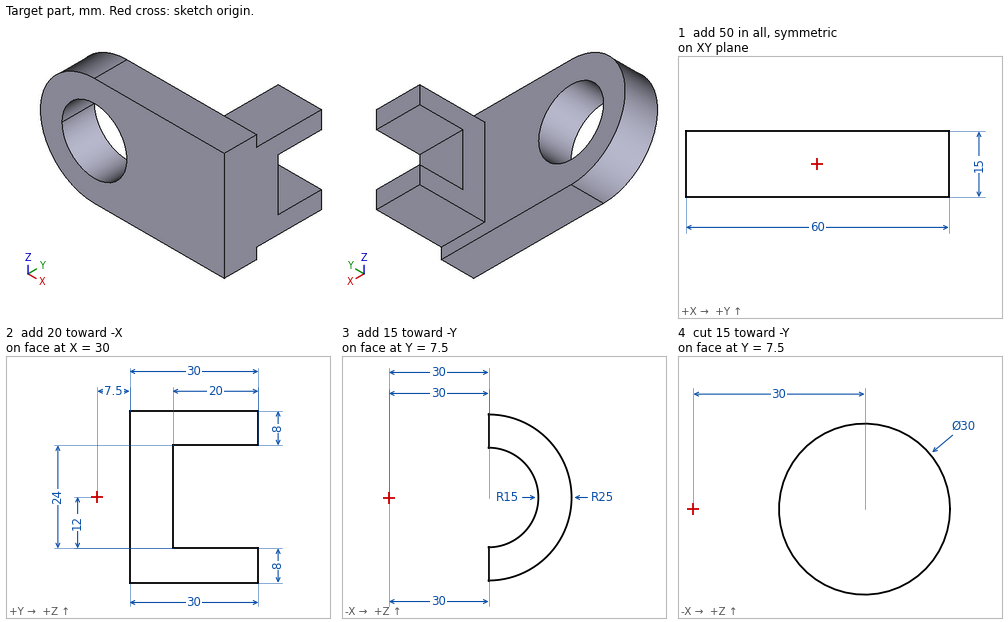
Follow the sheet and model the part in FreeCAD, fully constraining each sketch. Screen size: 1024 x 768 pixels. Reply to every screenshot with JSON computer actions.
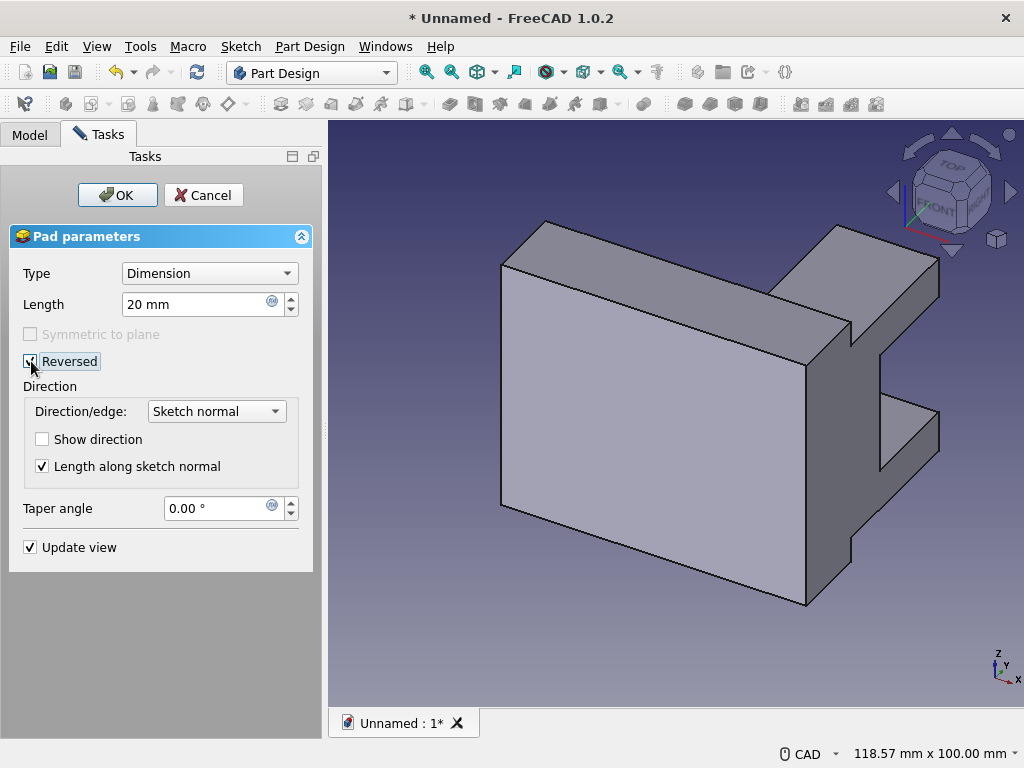
{"action": "left_click", "coordinate": [118, 195]}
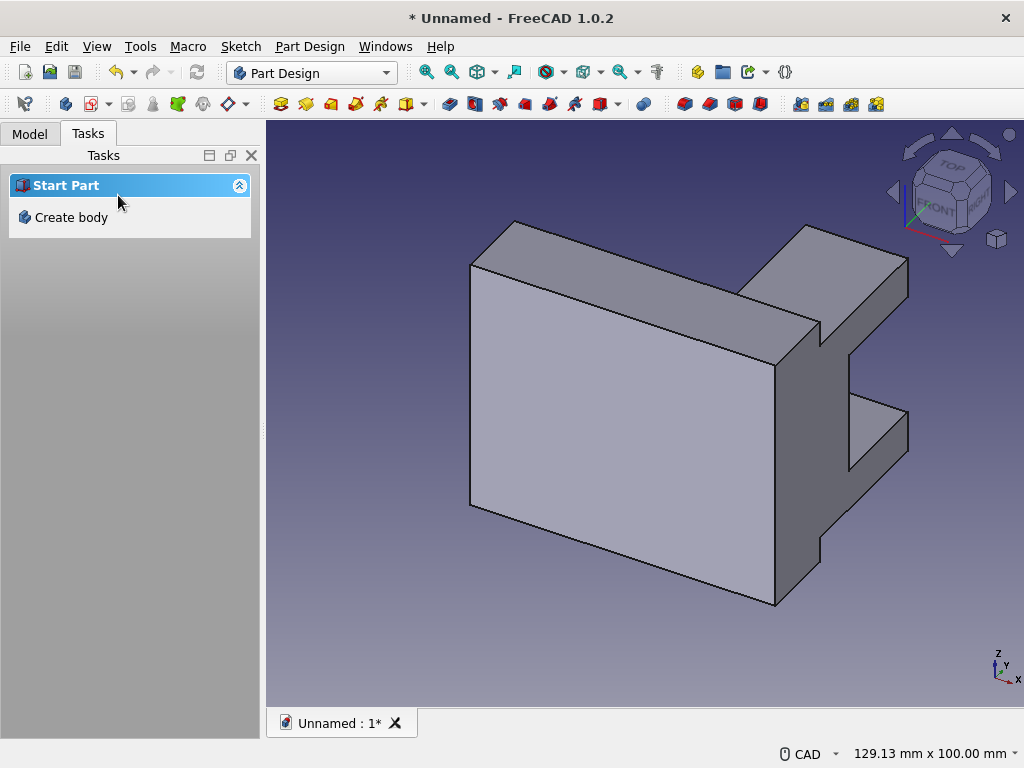
{"action": "key", "text": "4"}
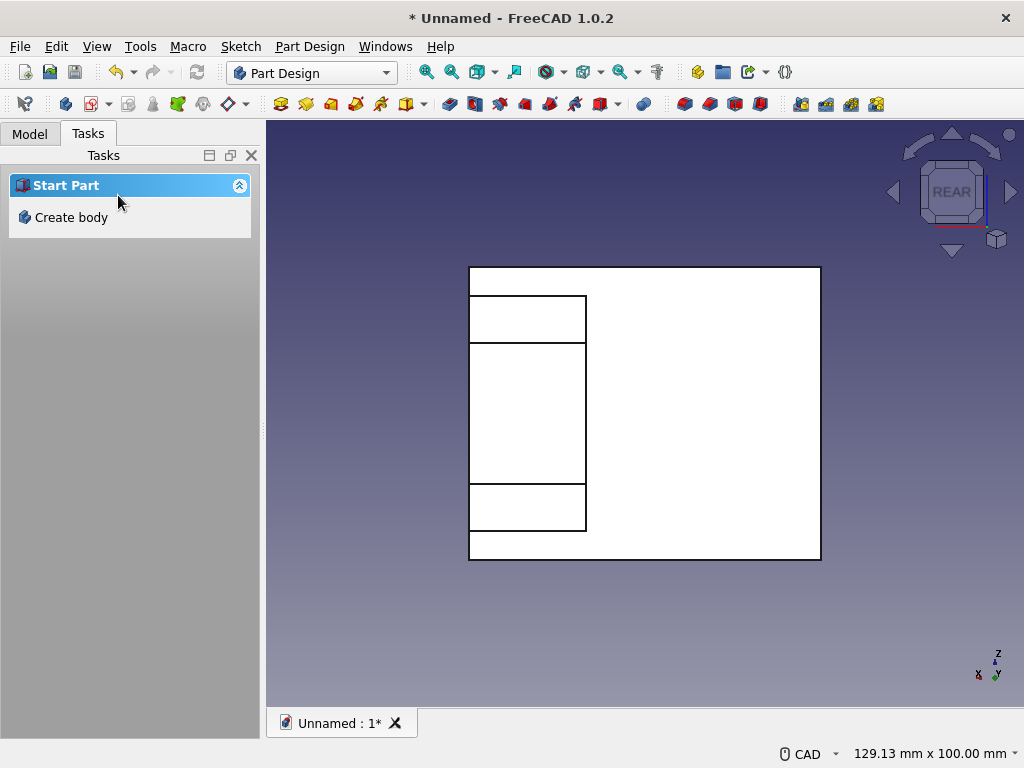
{"action": "left_click", "coordinate": [695, 412]}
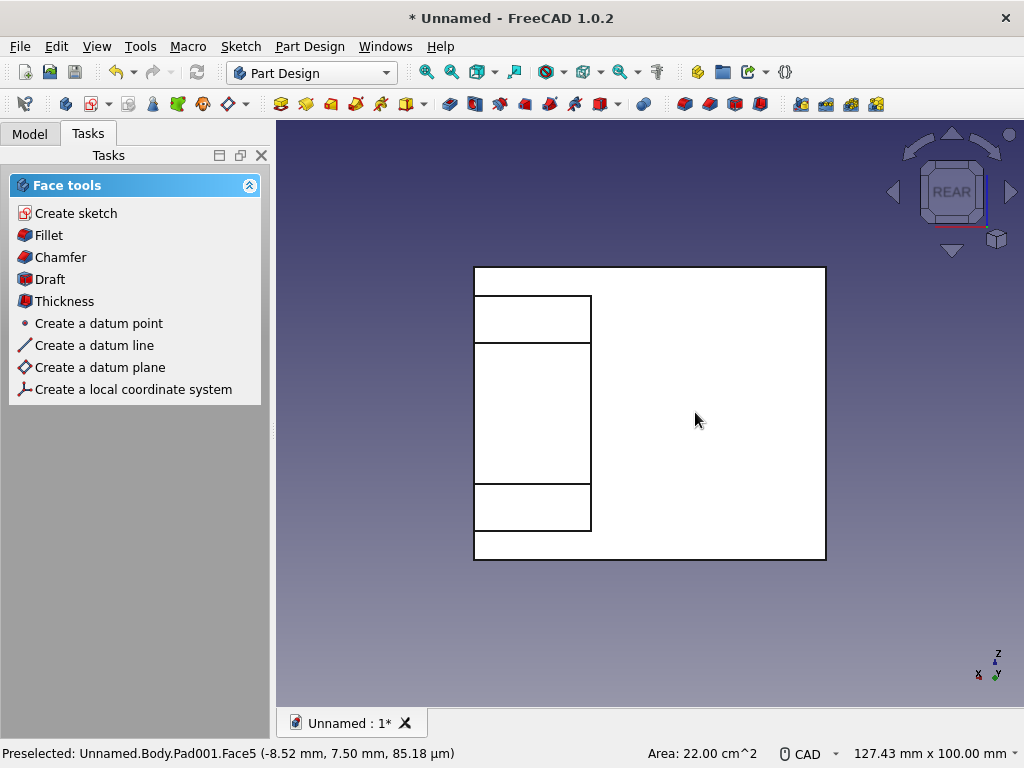
{"action": "left_click", "coordinate": [90, 104]}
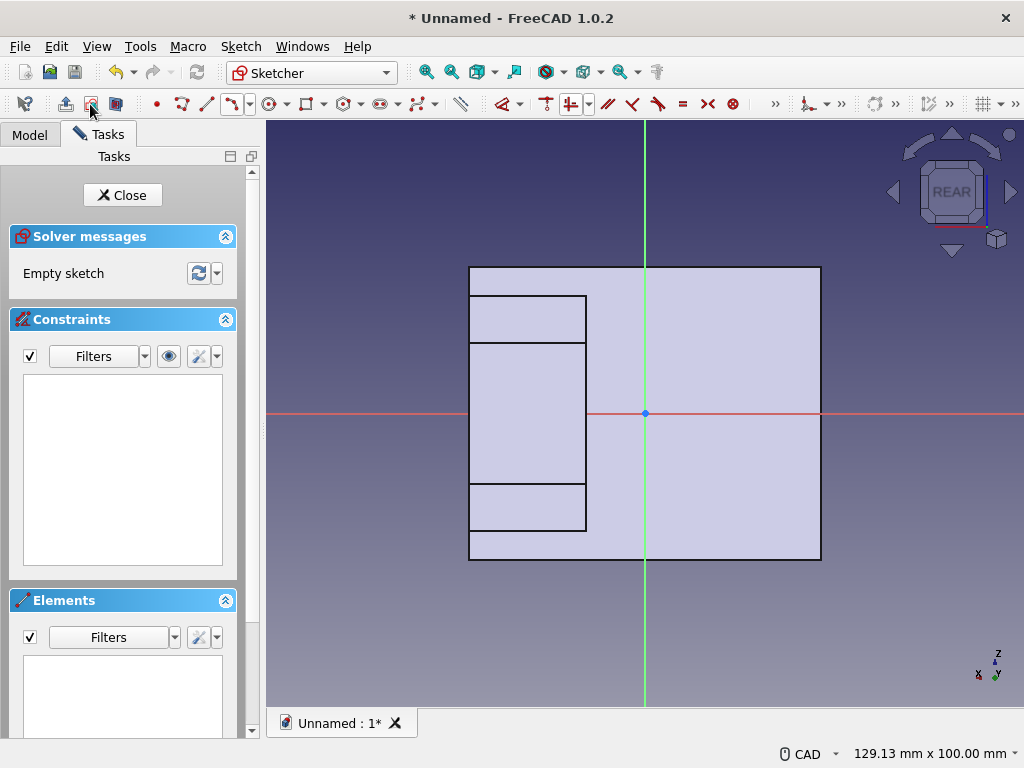
{"action": "scroll", "coordinate": [294, 414], "scroll_direction": "down", "scroll_amount": 2}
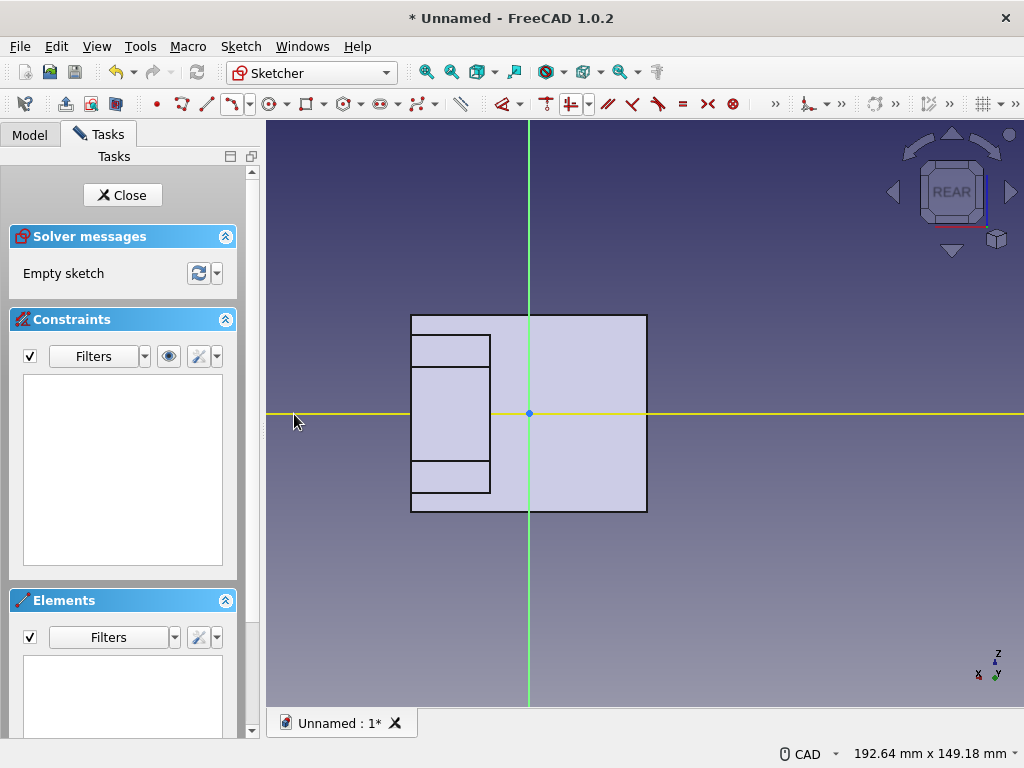
{"action": "scroll", "coordinate": [712, 414], "scroll_direction": "up", "scroll_amount": 3}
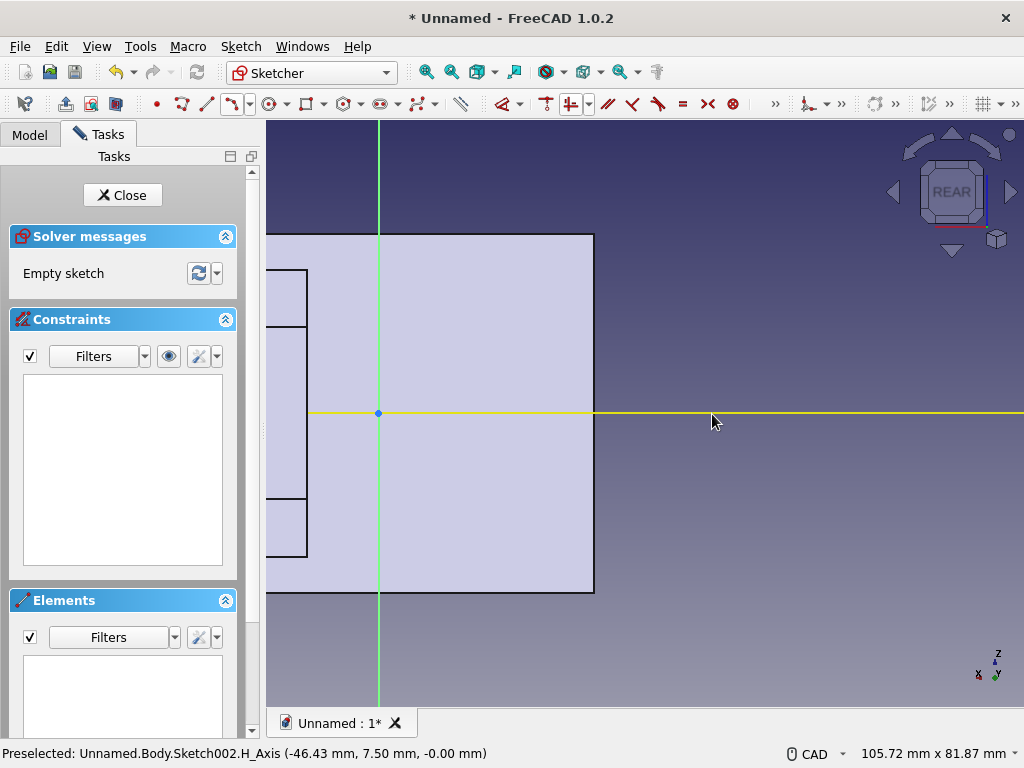
{"action": "key", "text": "g l"}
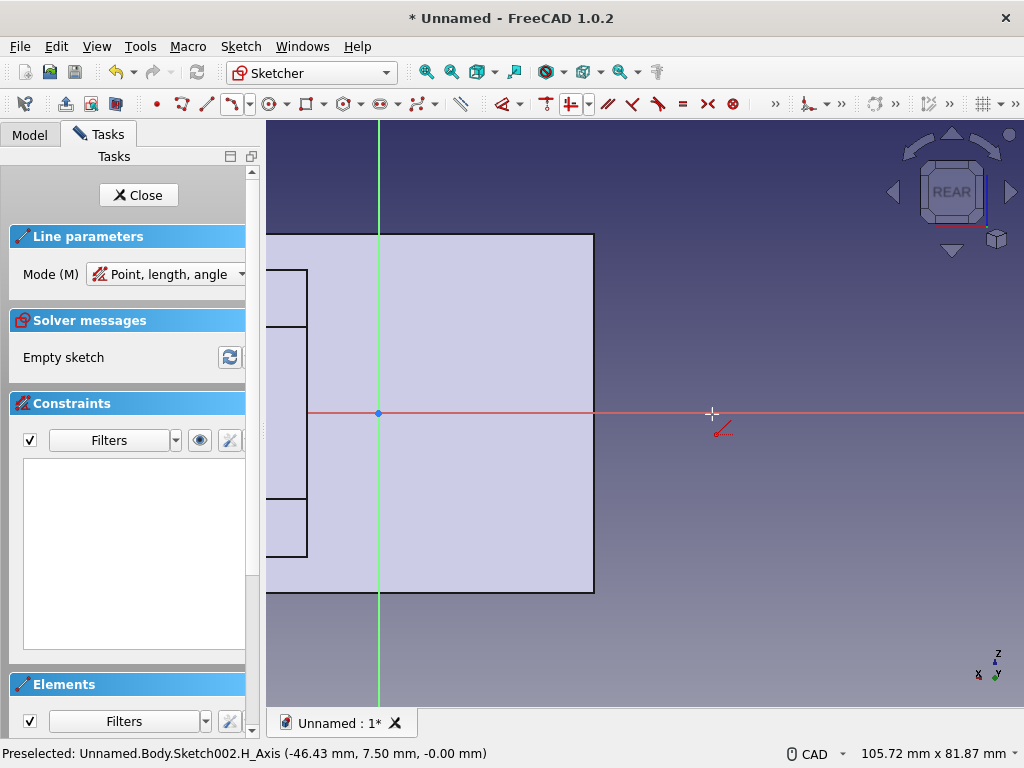
{"action": "left_click", "coordinate": [594, 521]}
{"action": "left_click", "coordinate": [594, 593]}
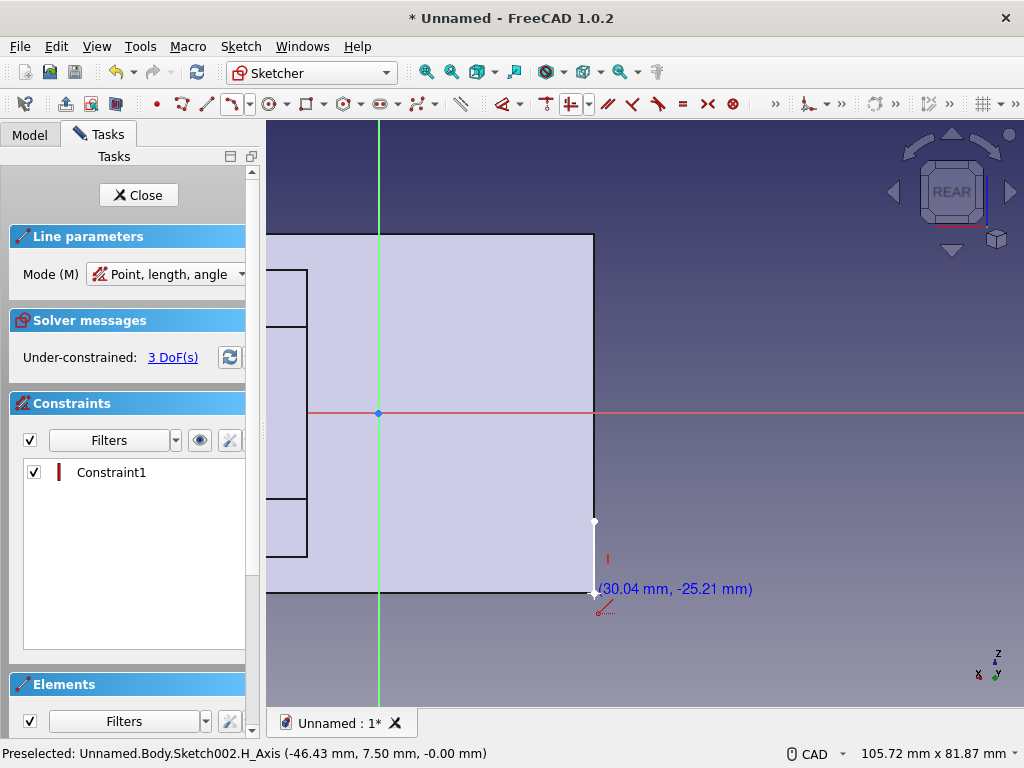
{"action": "left_click", "coordinate": [594, 234]}
{"action": "left_click", "coordinate": [594, 306]}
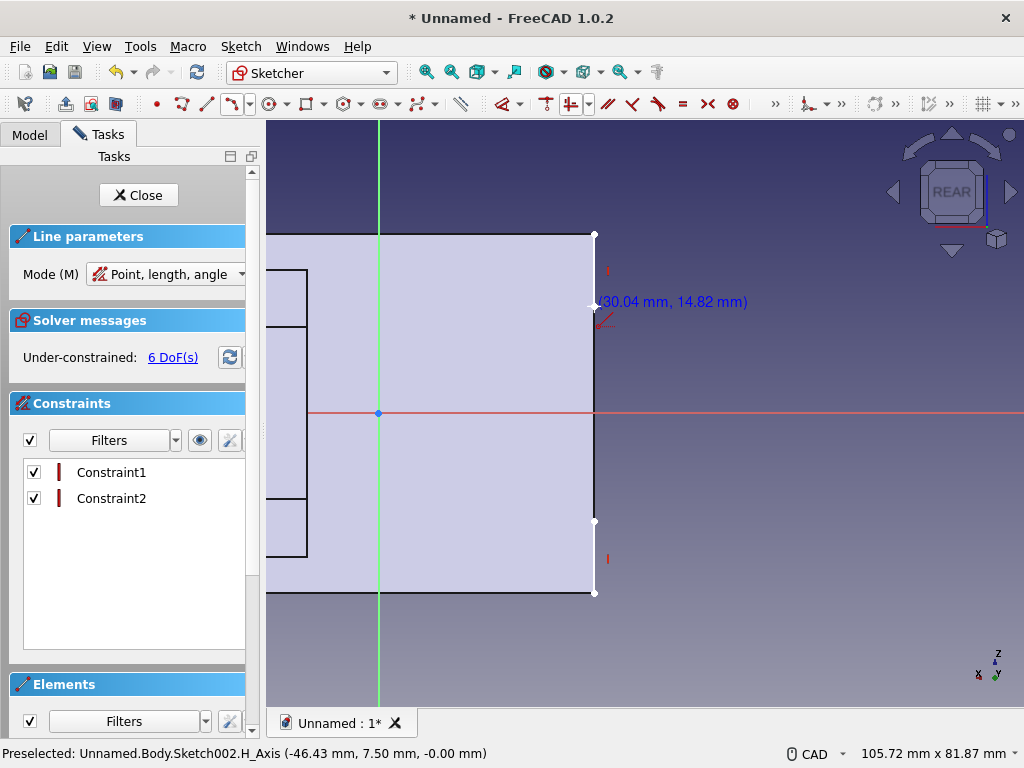
{"action": "left_click", "coordinate": [232, 104]}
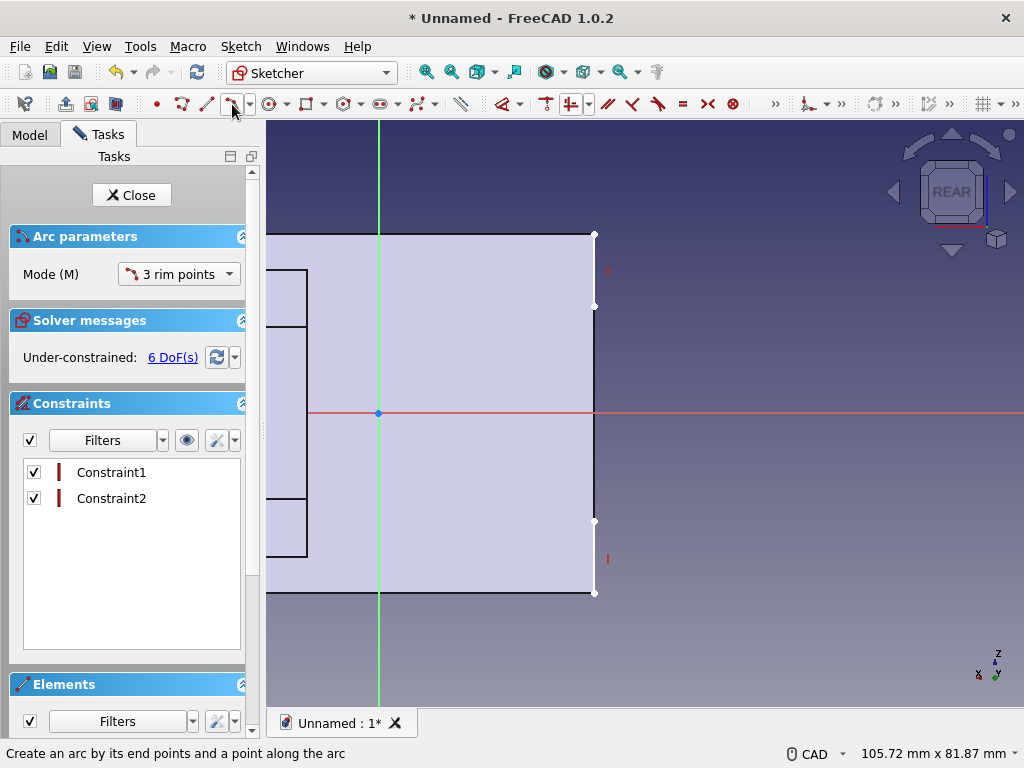
{"action": "left_click", "coordinate": [594, 594]}
{"action": "left_click", "coordinate": [594, 235]}
{"action": "left_click", "coordinate": [764, 469]}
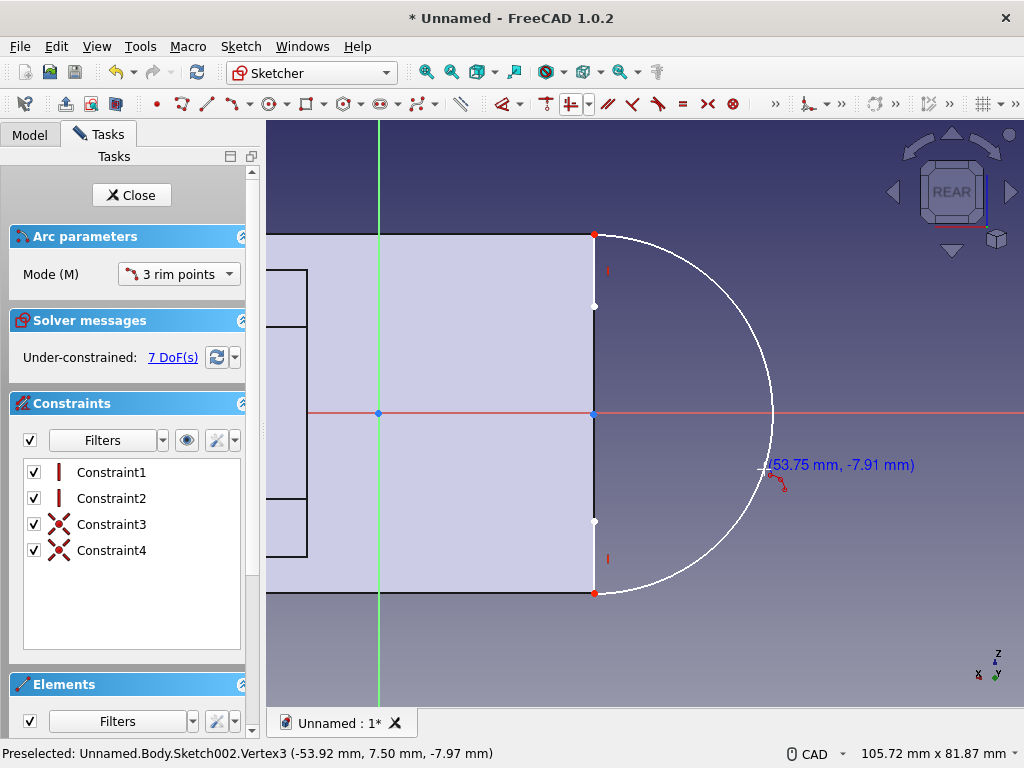
{"action": "left_click", "coordinate": [594, 307]}
{"action": "left_click", "coordinate": [594, 522]}
{"action": "left_click", "coordinate": [696, 447]}
{"action": "key", "text": "Escape"}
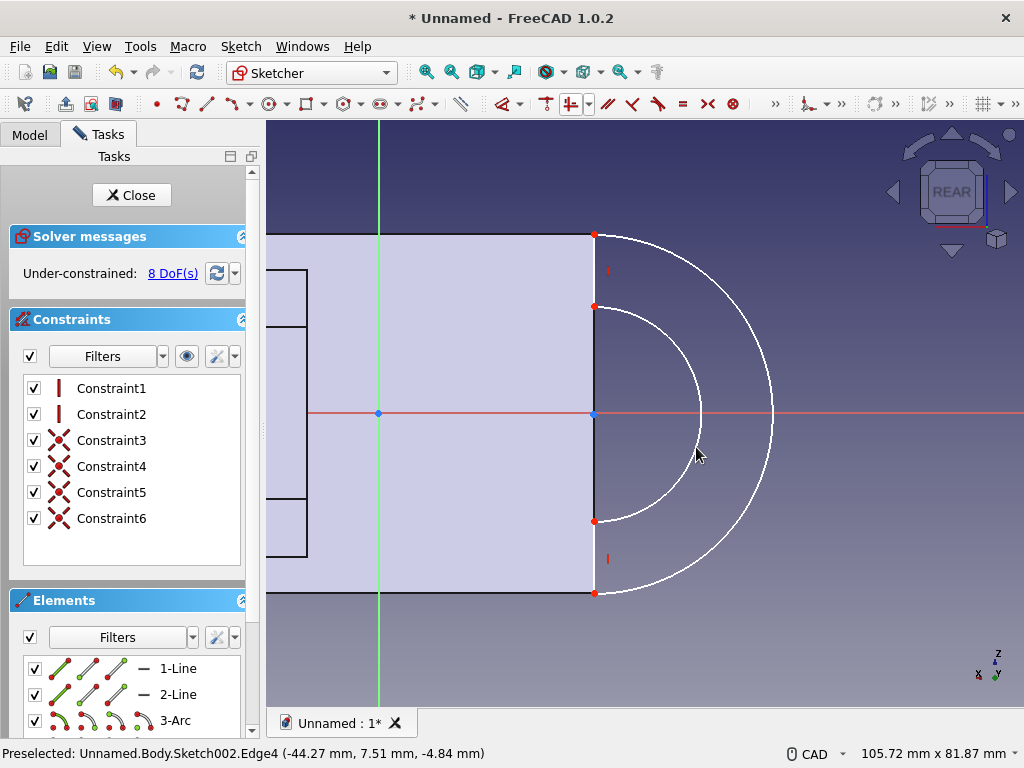
{"action": "left_click", "coordinate": [739, 520]}